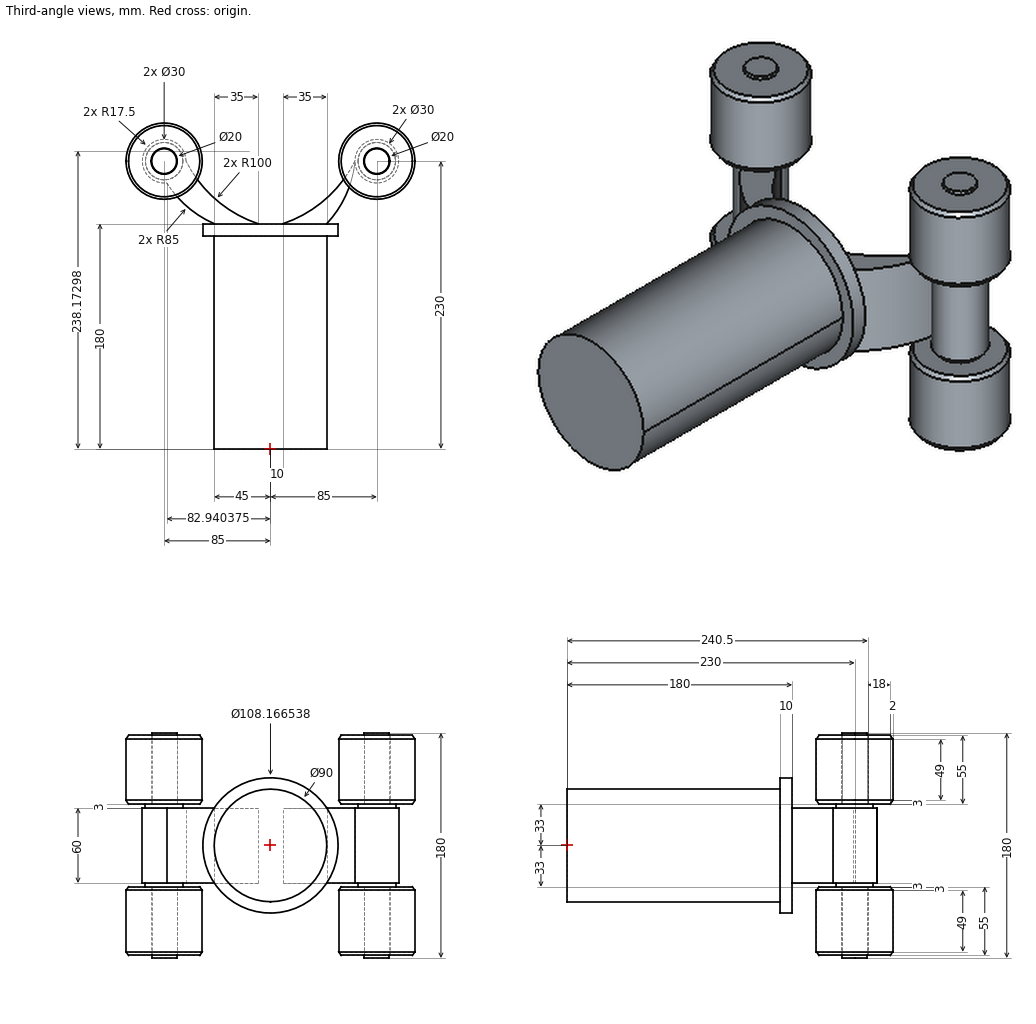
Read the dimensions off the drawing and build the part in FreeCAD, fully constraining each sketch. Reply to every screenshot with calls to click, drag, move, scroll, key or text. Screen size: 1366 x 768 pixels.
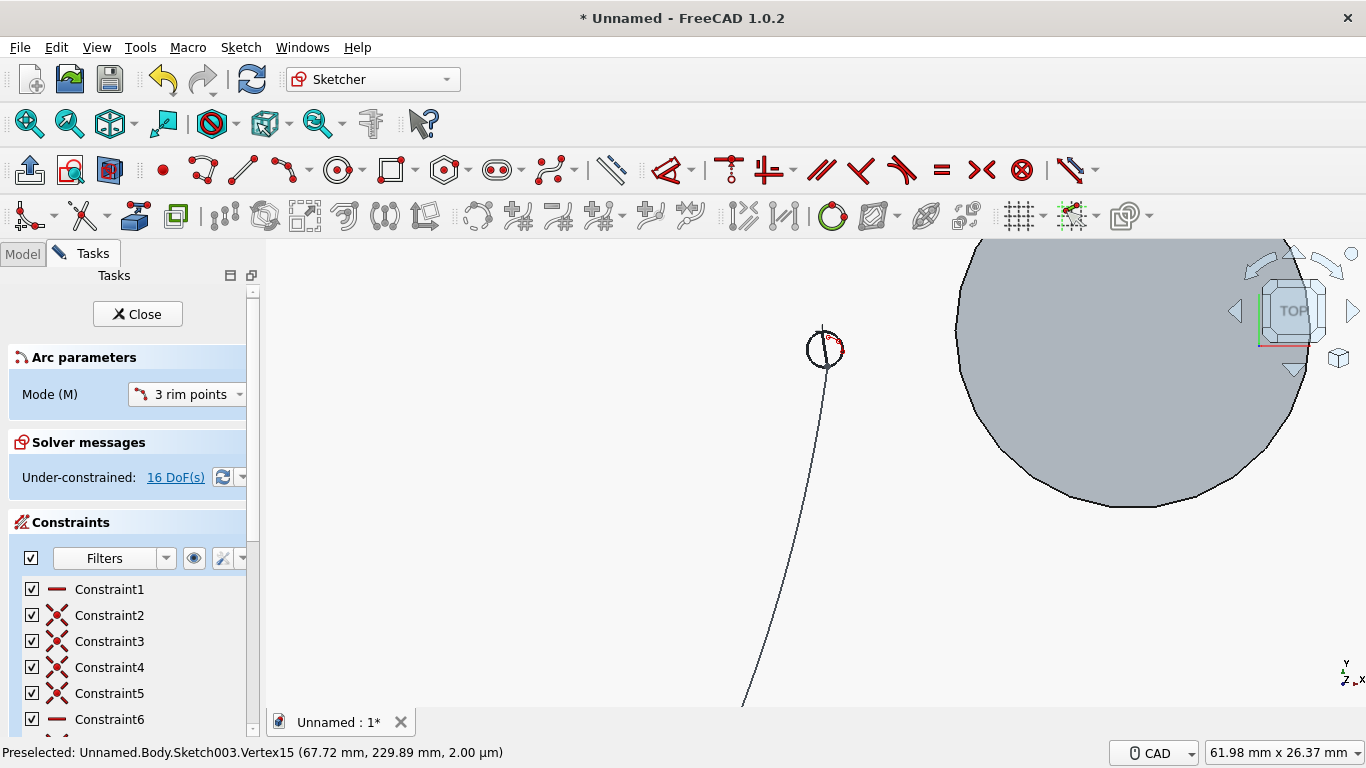
scroll(834, 329, down, 13)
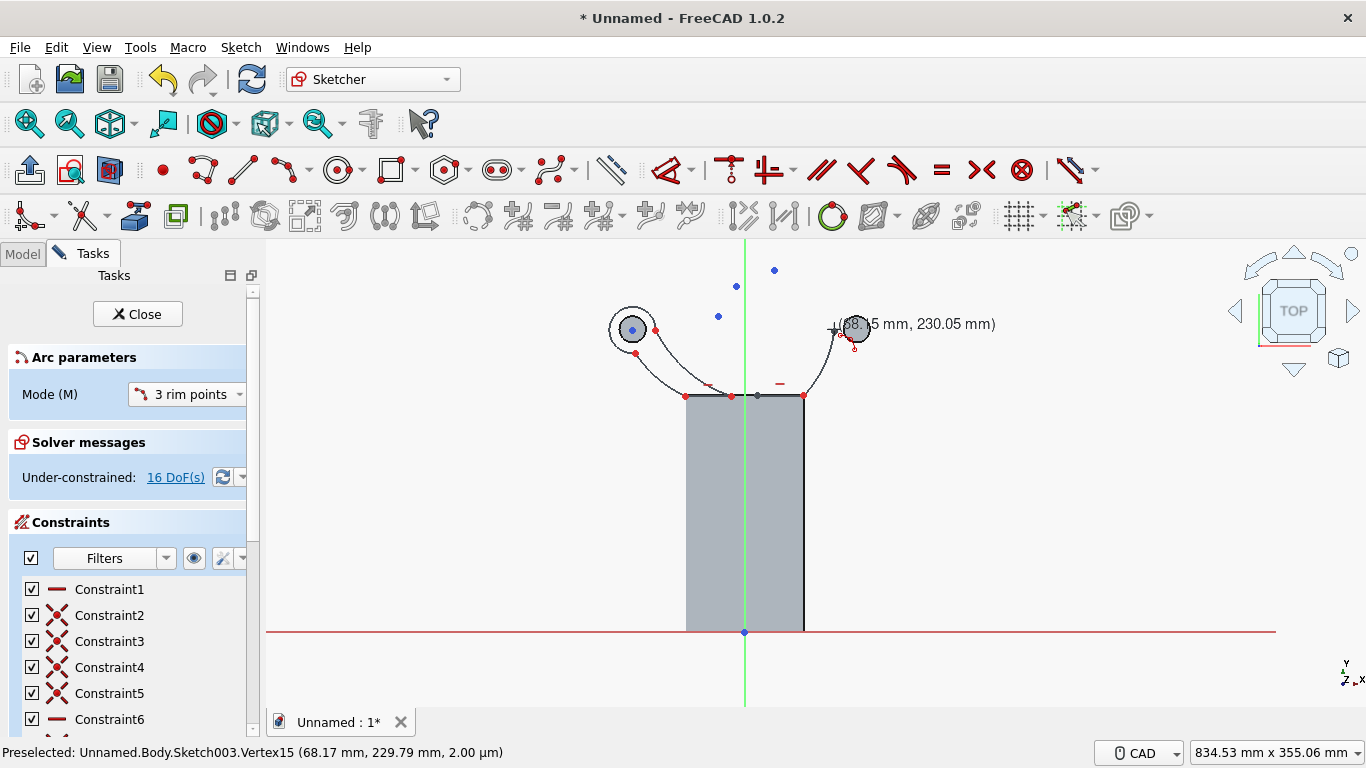
click(880, 329)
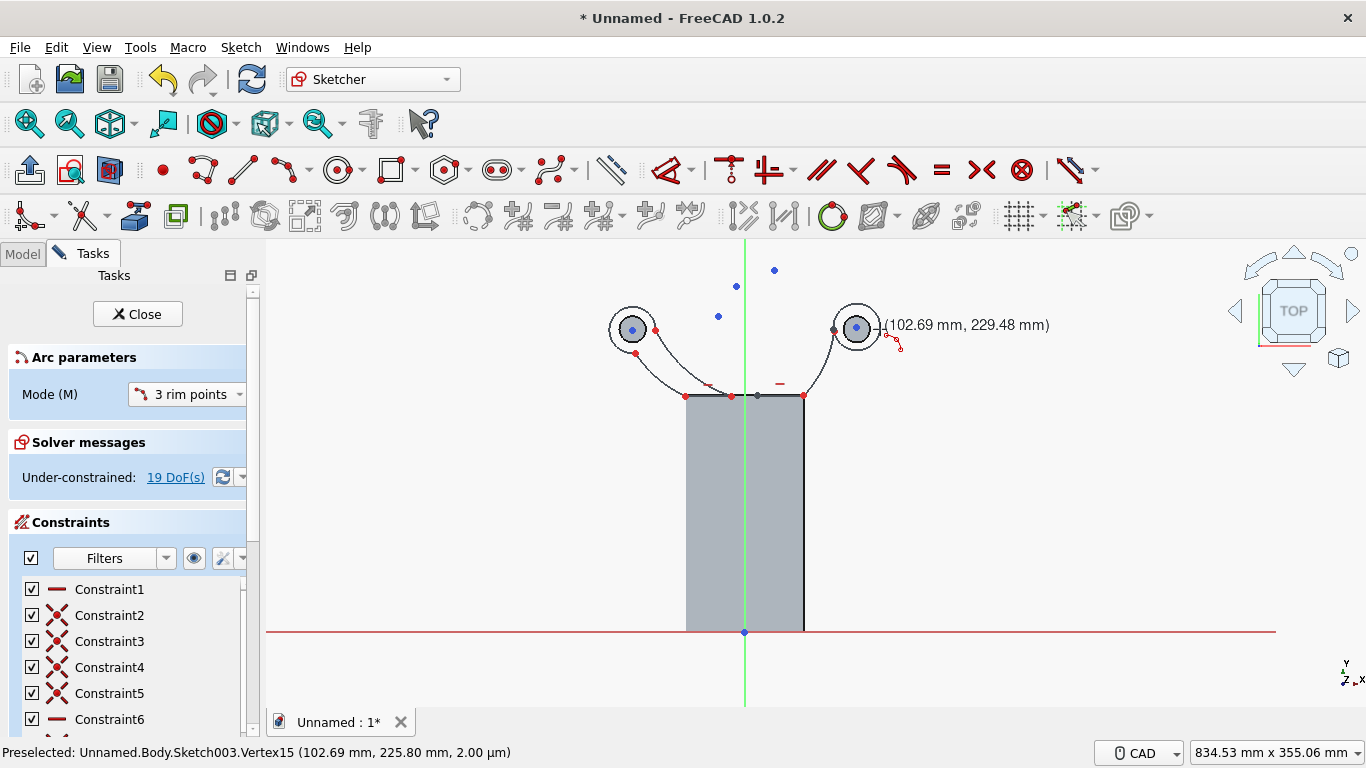
scroll(834, 329, up, 13)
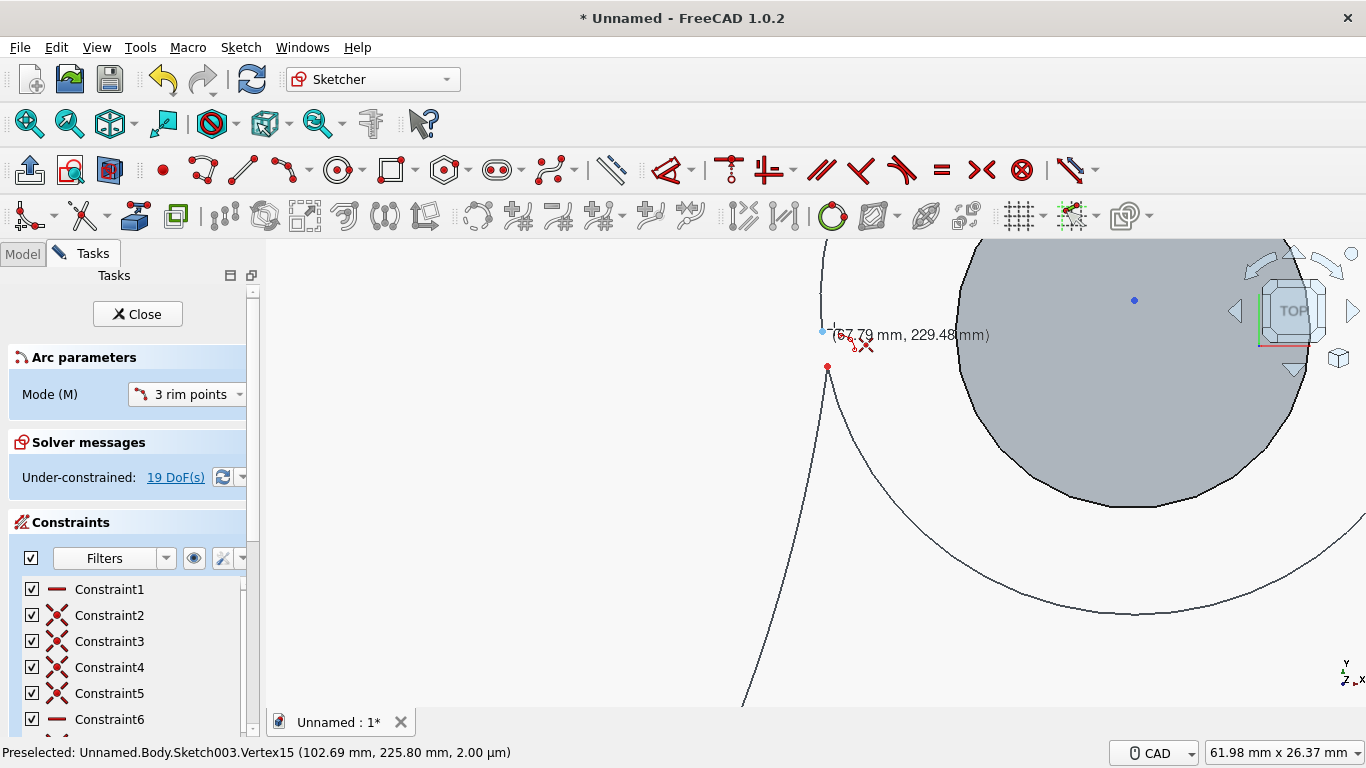
click(822, 332)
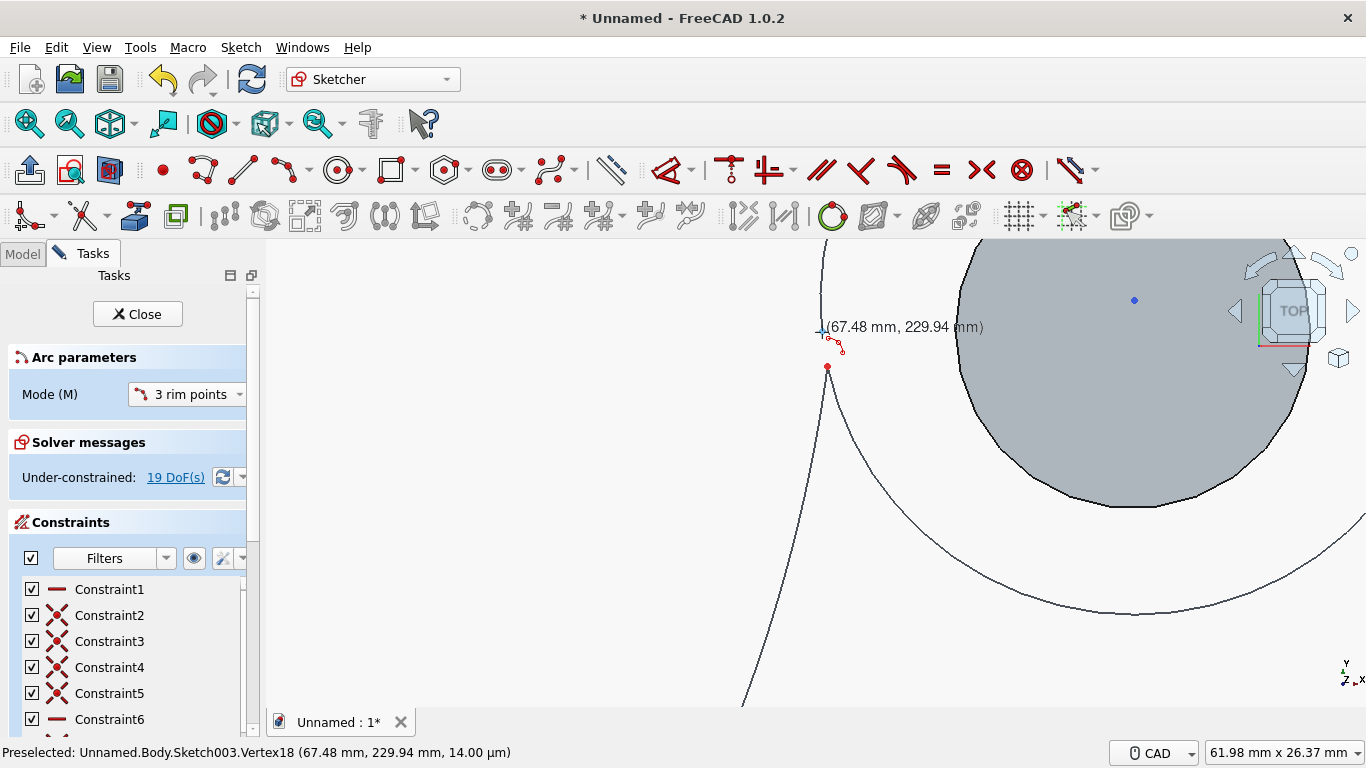
scroll(834, 329, down, 13)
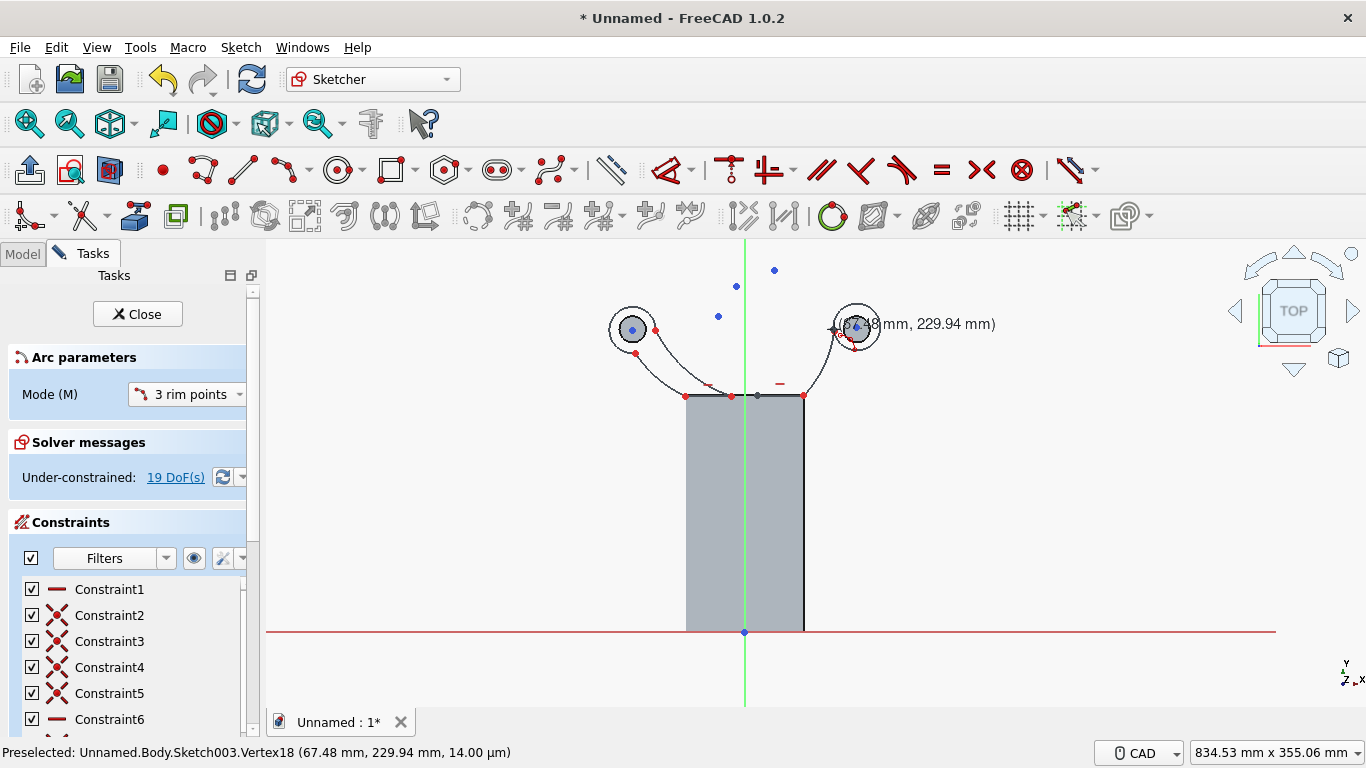
click(758, 396)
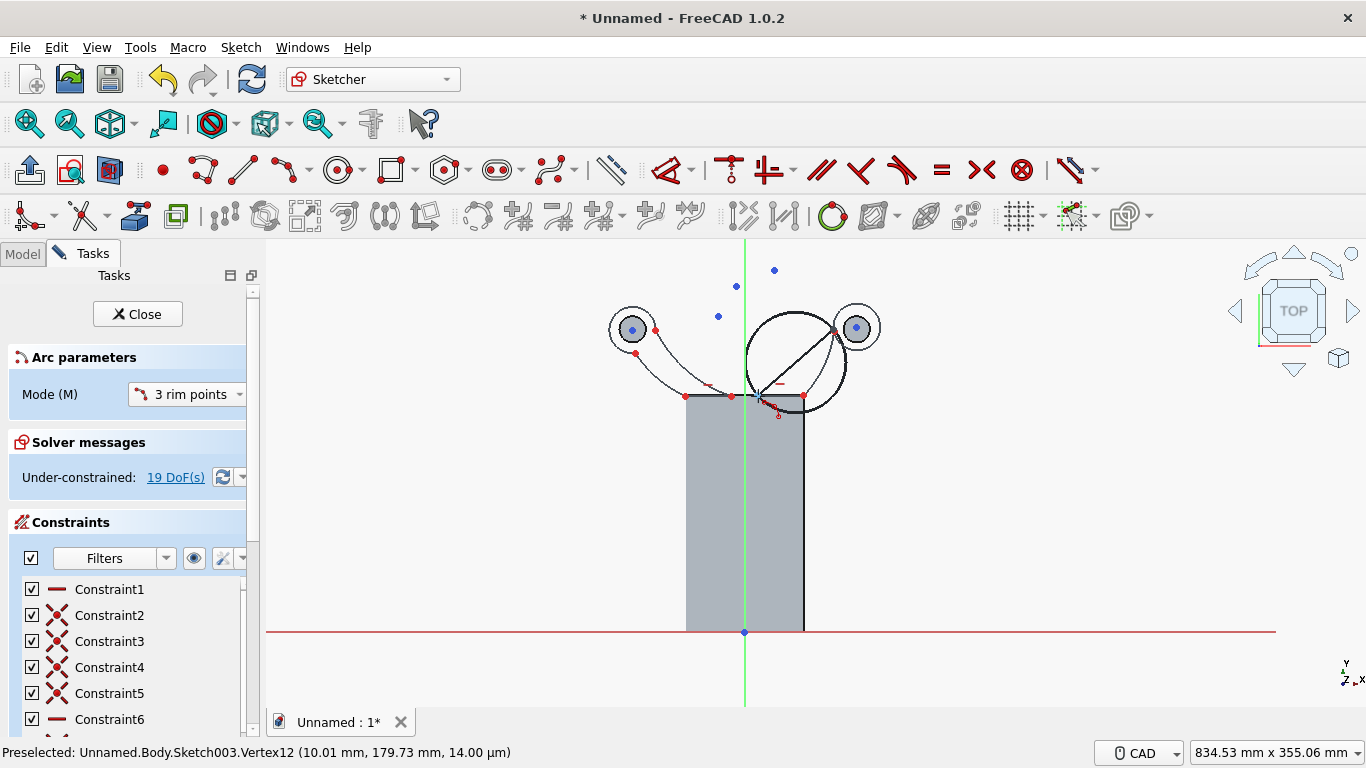
scroll(802, 370, up, 3)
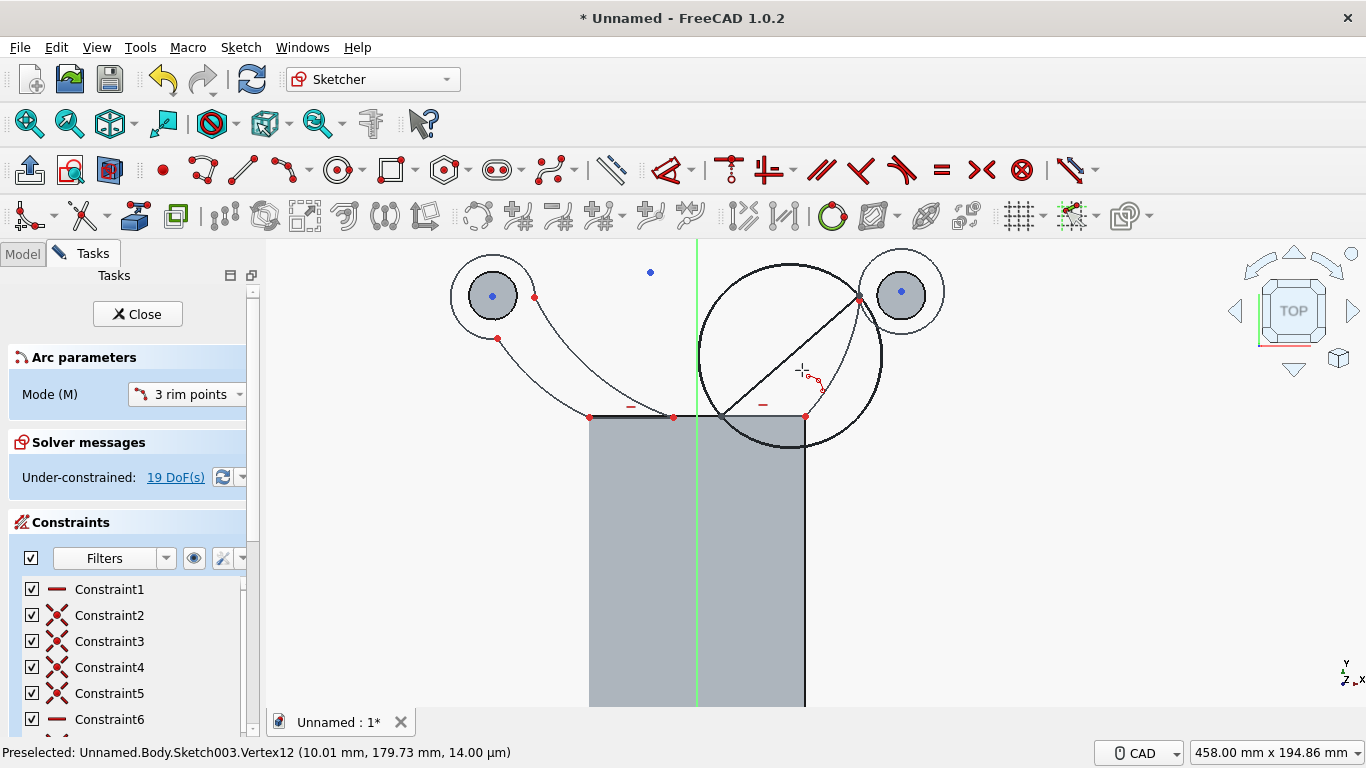
click(802, 369)
key(Escape)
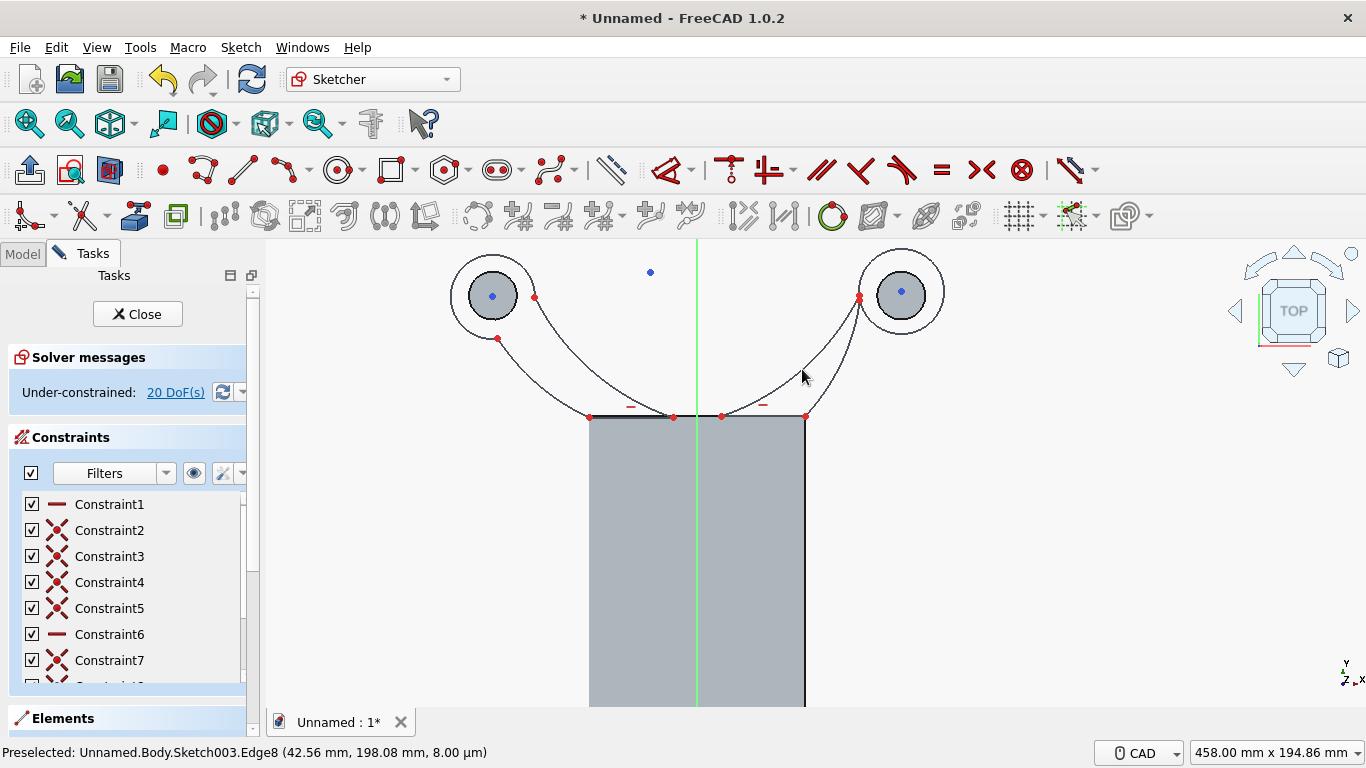
click(520, 368)